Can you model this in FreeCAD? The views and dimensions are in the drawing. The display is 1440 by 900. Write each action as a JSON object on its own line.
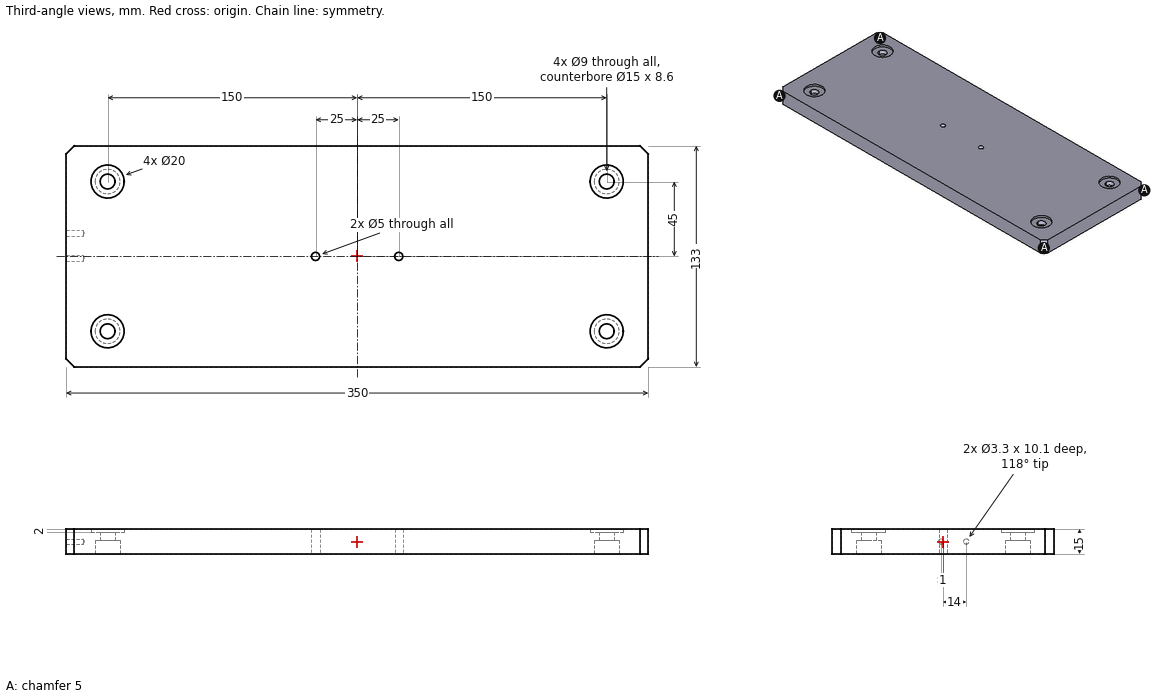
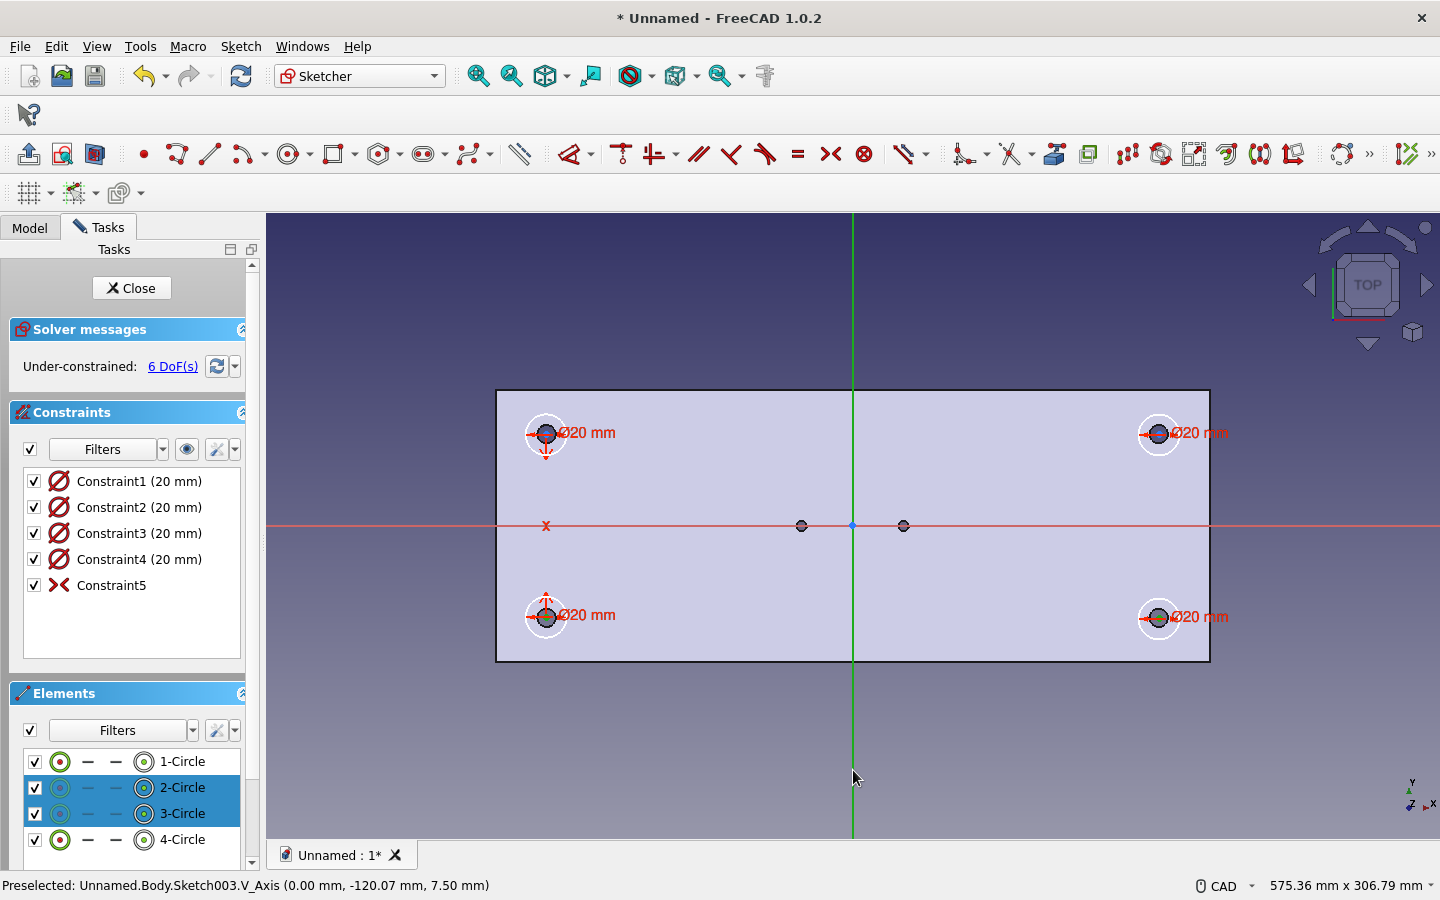
{"action": "key", "text": "s"}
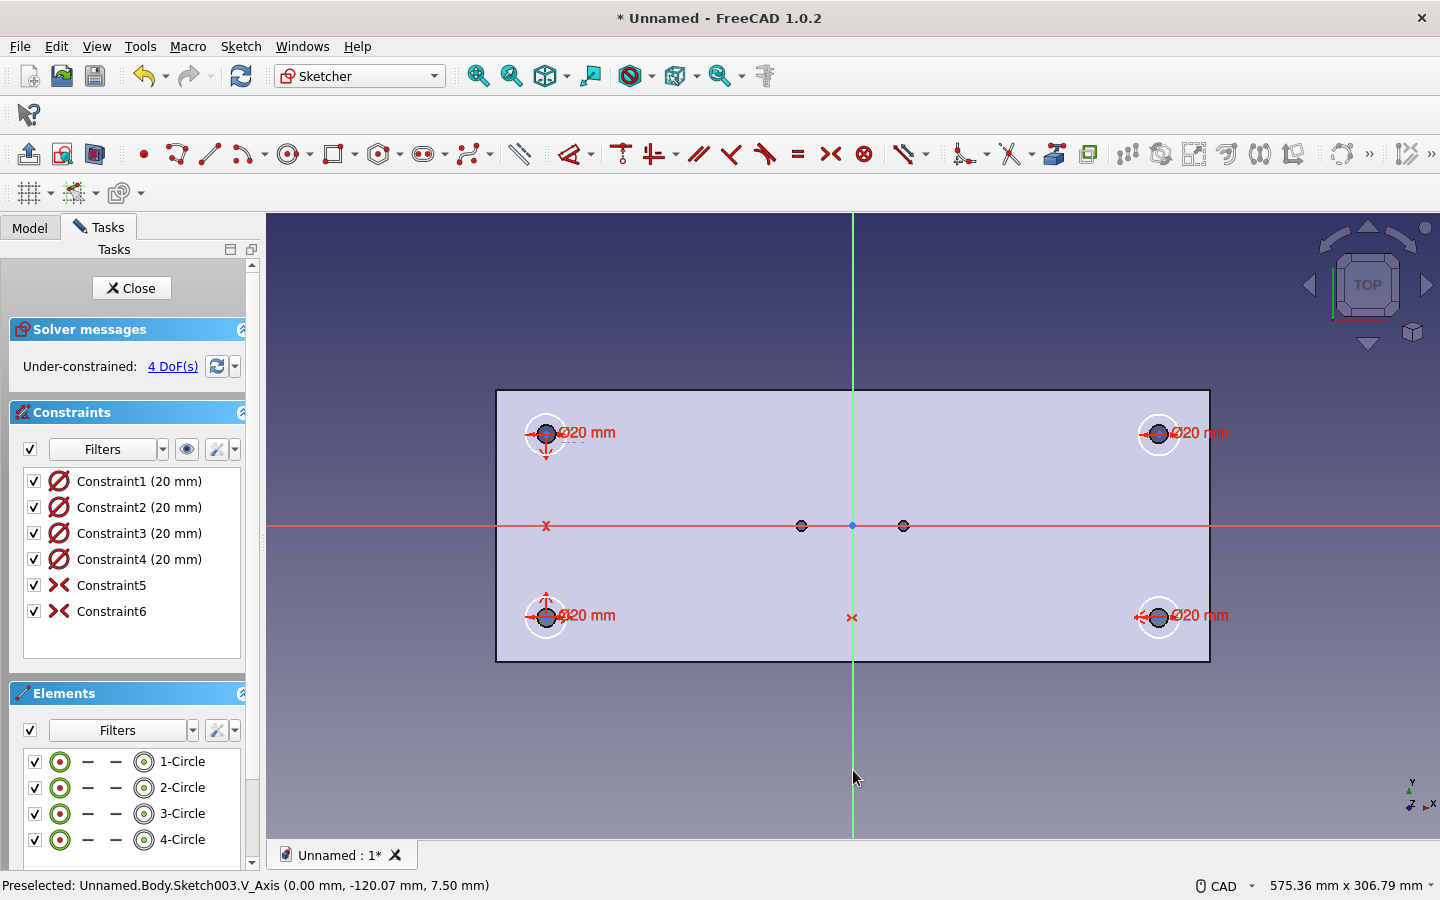
{"action": "left_click", "coordinate": [546, 435]}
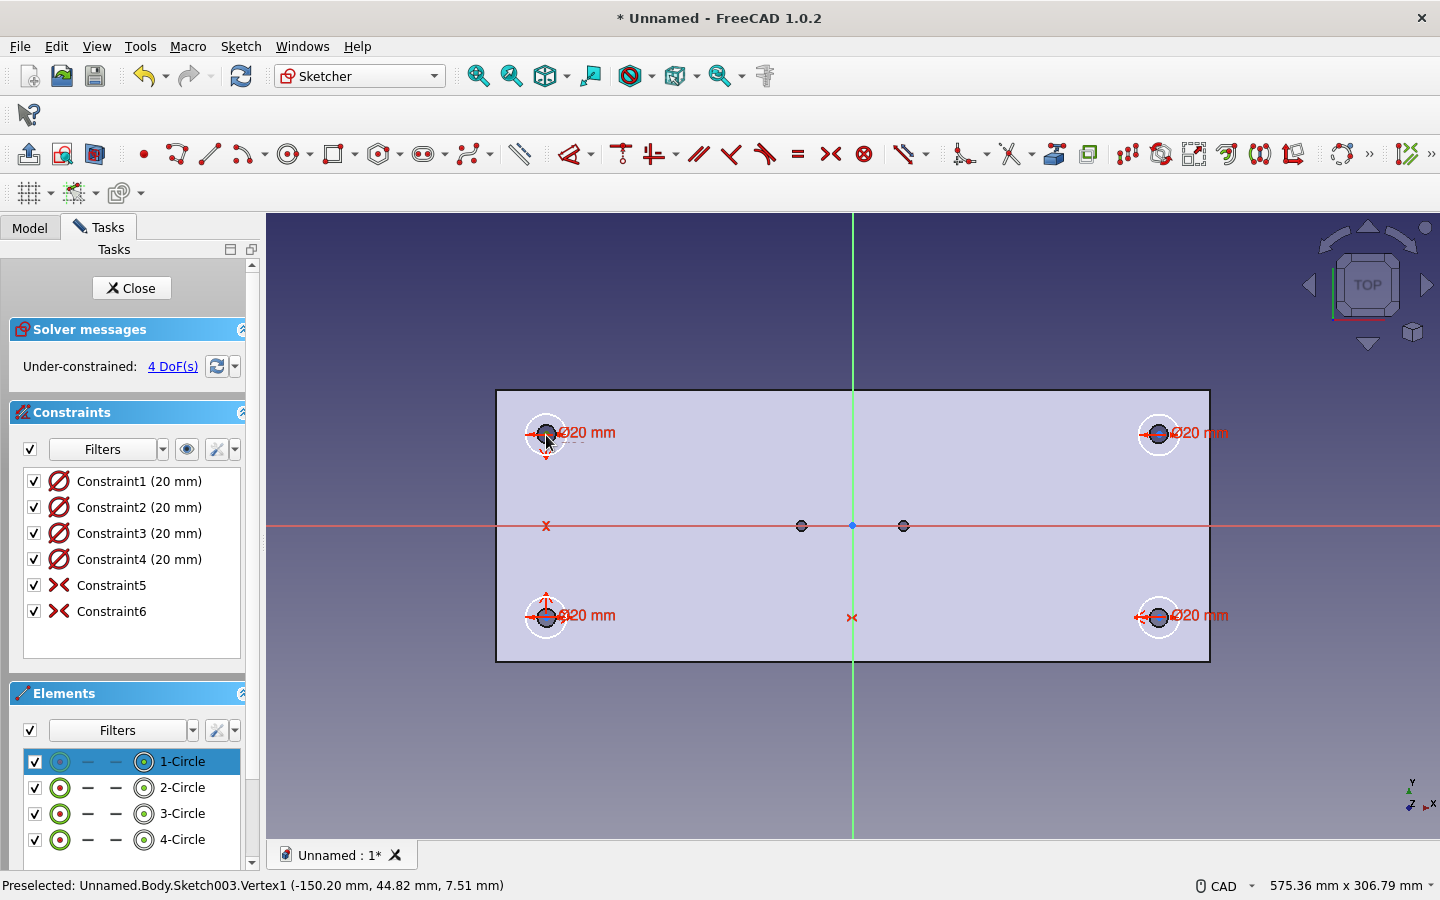
{"action": "left_click", "coordinate": [1159, 435]}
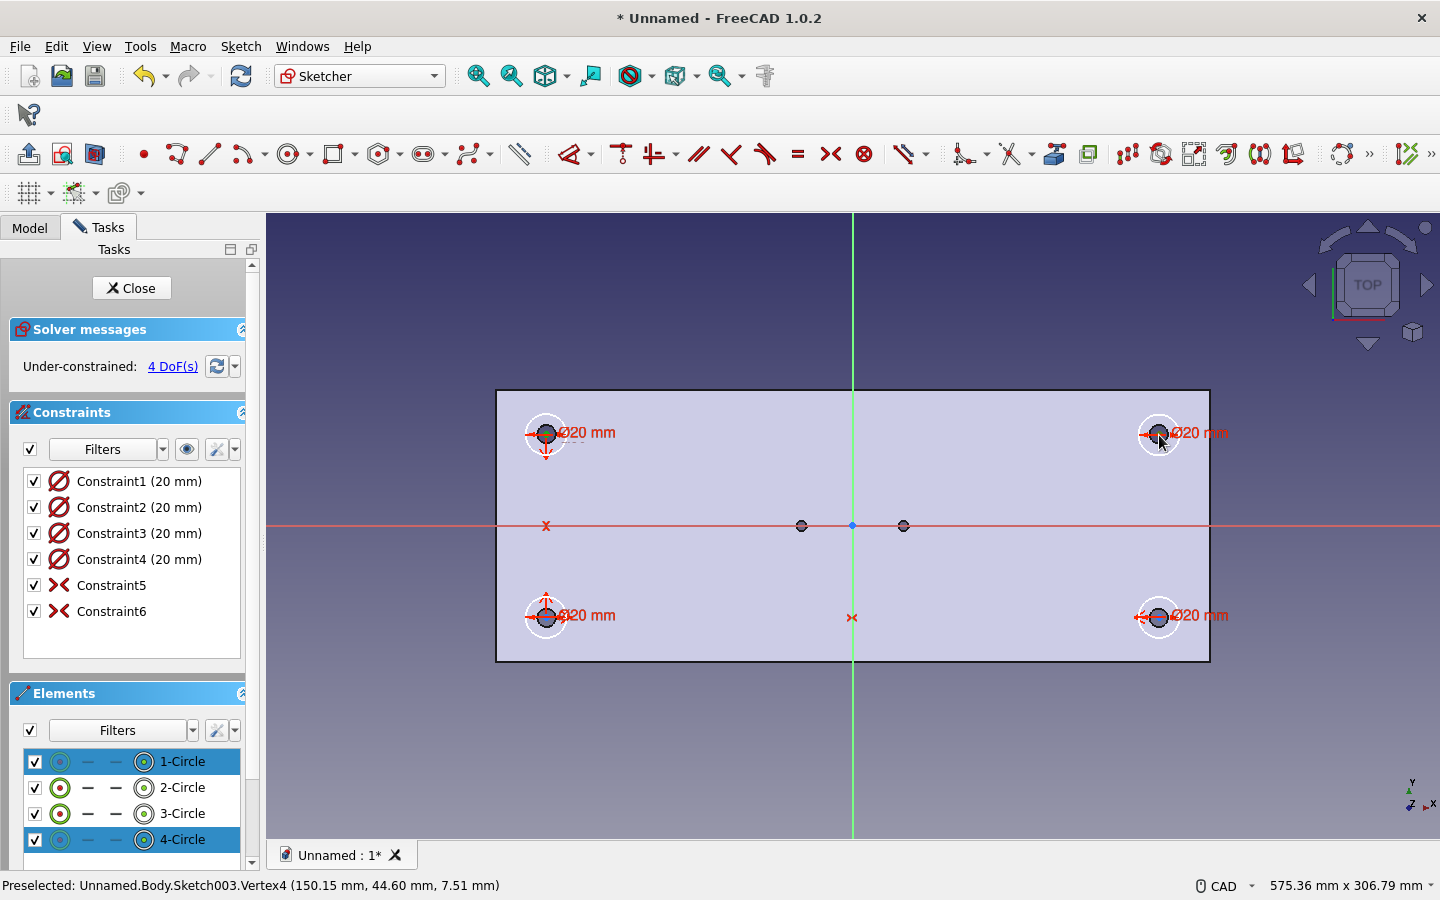
{"action": "left_click", "coordinate": [853, 770]}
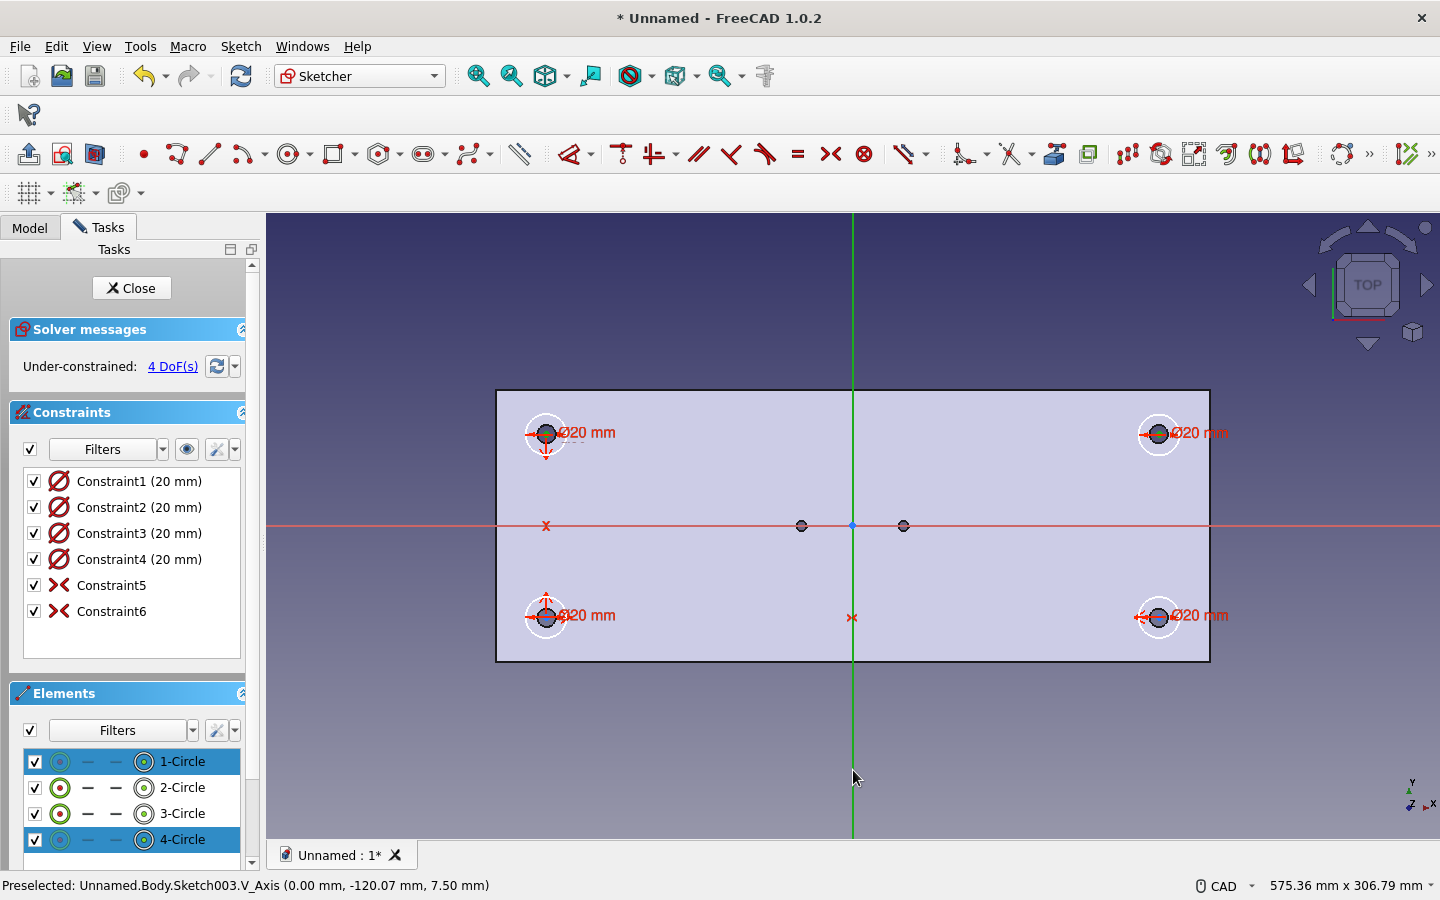
{"action": "key", "text": "s"}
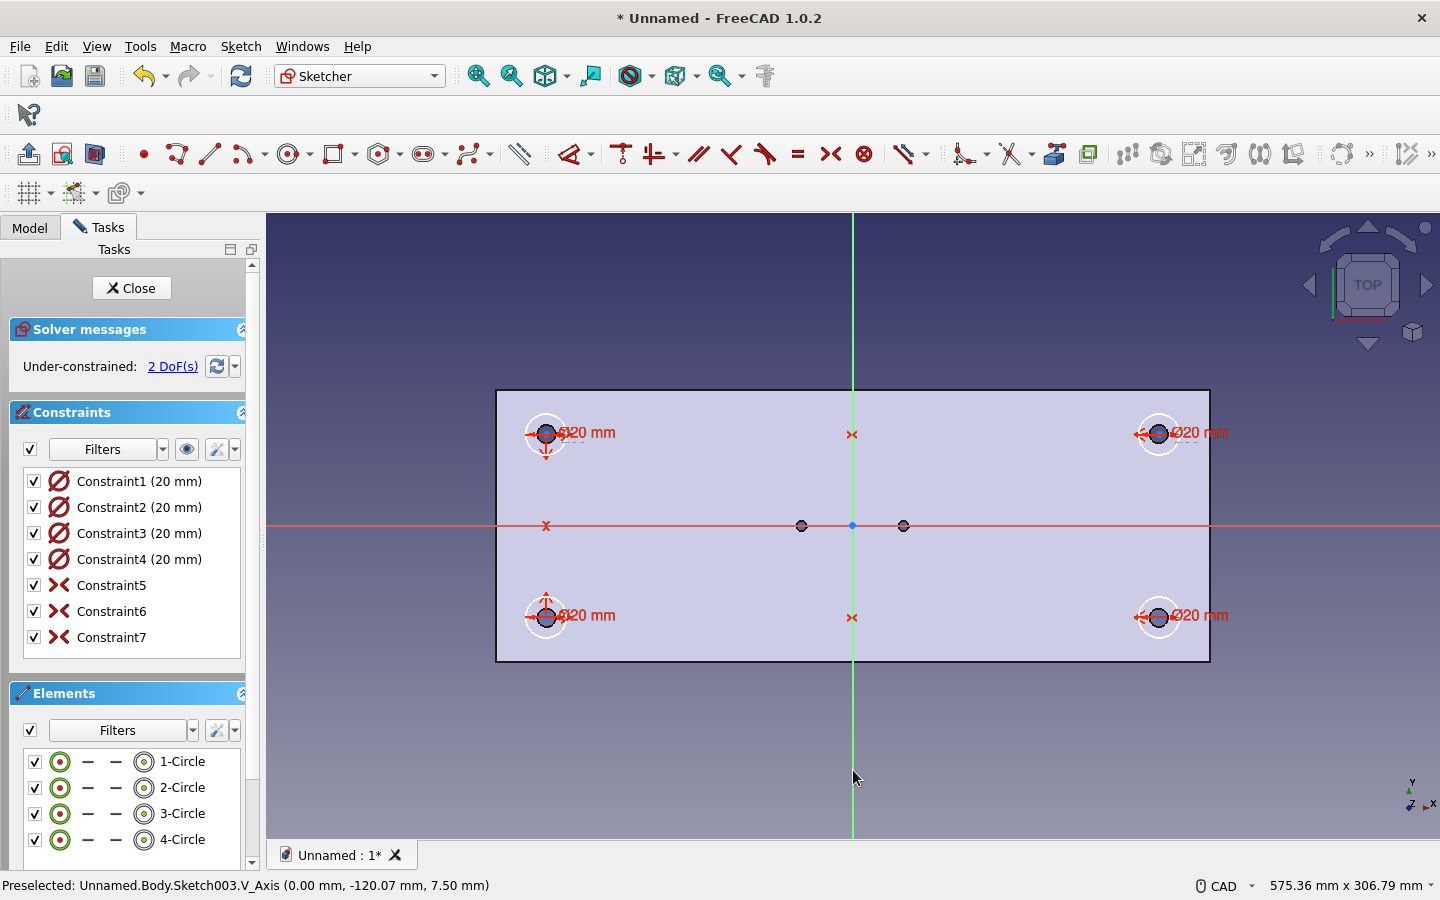
{"action": "key", "text": "d"}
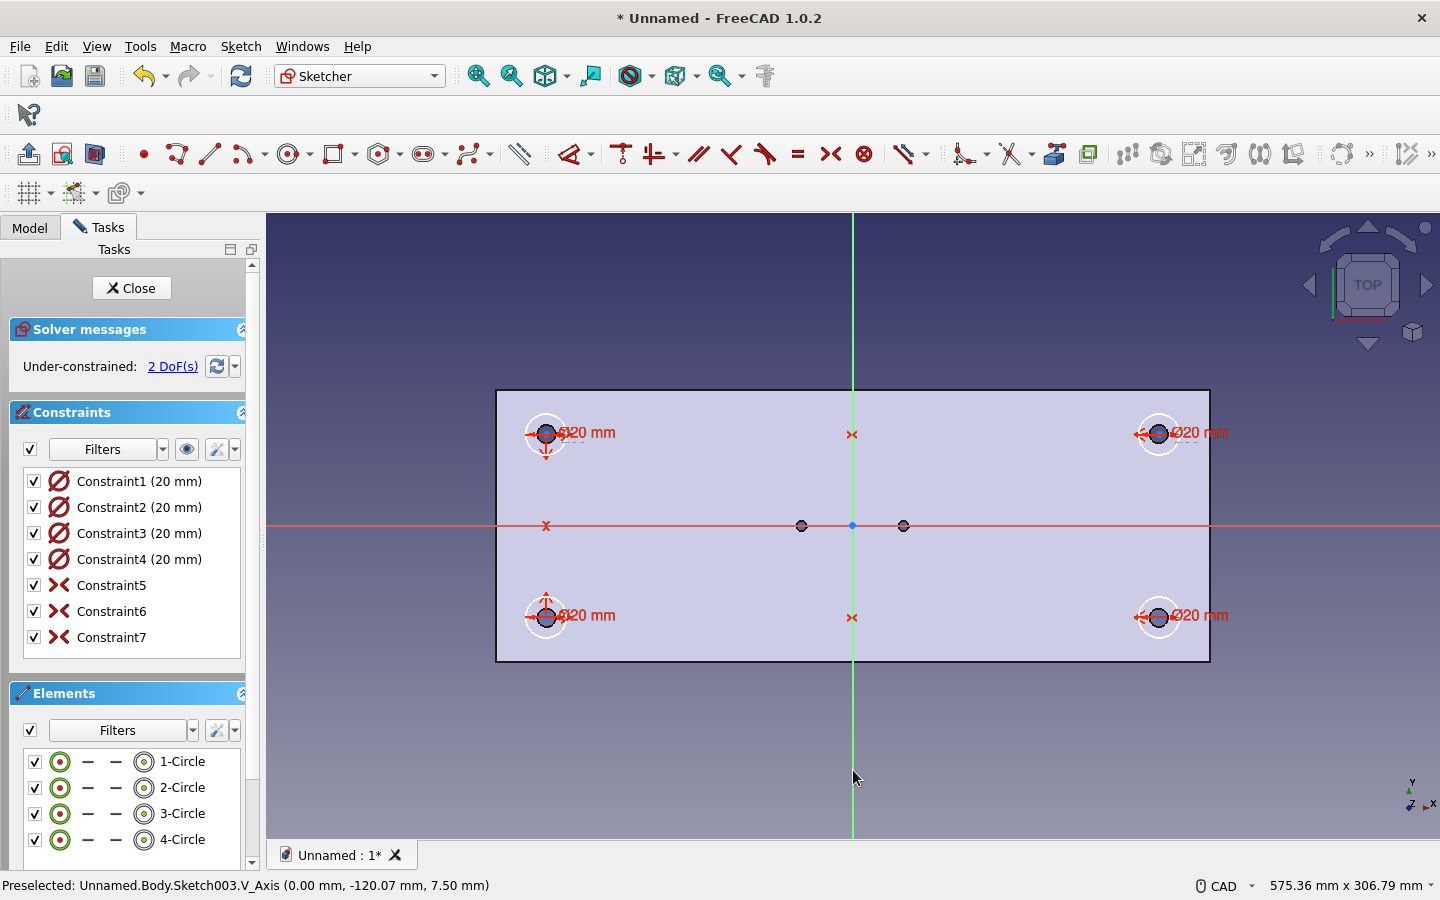
{"action": "left_click", "coordinate": [546, 435]}
{"action": "left_click", "coordinate": [512, 480]}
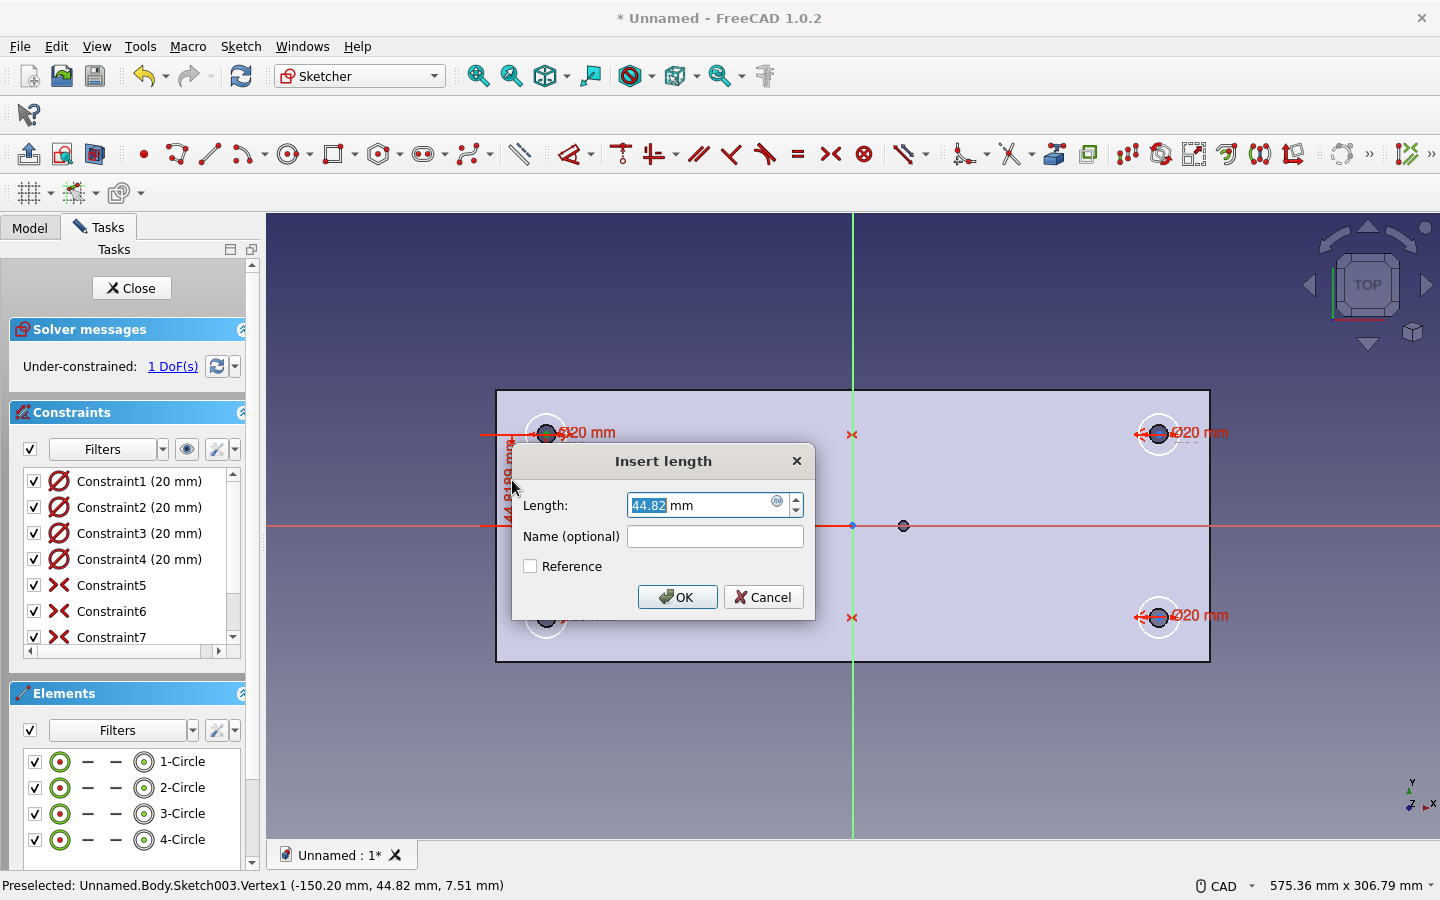
{"action": "type", "text": "45"}
{"action": "key", "text": "Return"}